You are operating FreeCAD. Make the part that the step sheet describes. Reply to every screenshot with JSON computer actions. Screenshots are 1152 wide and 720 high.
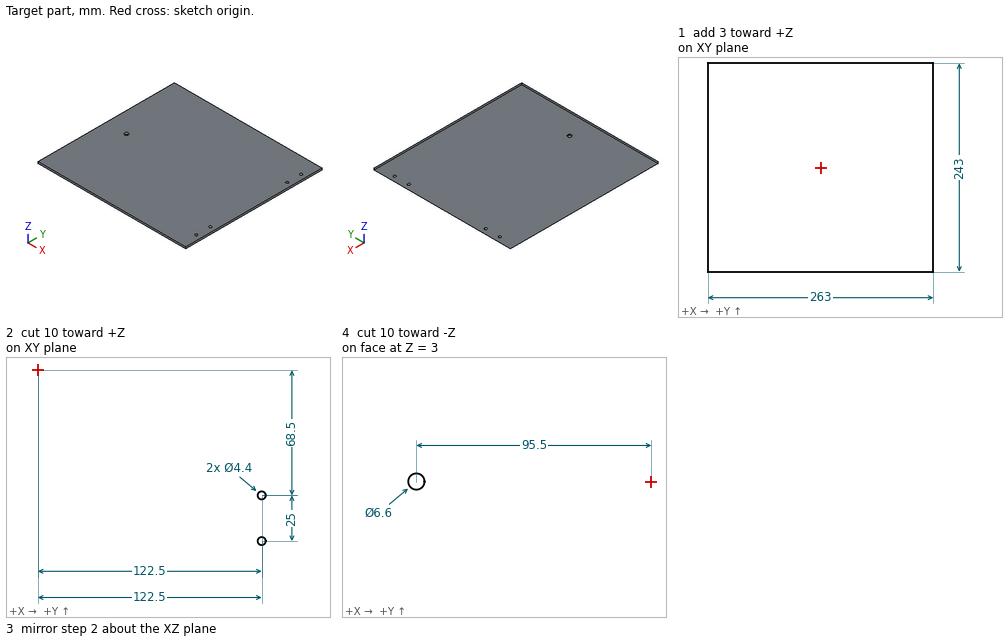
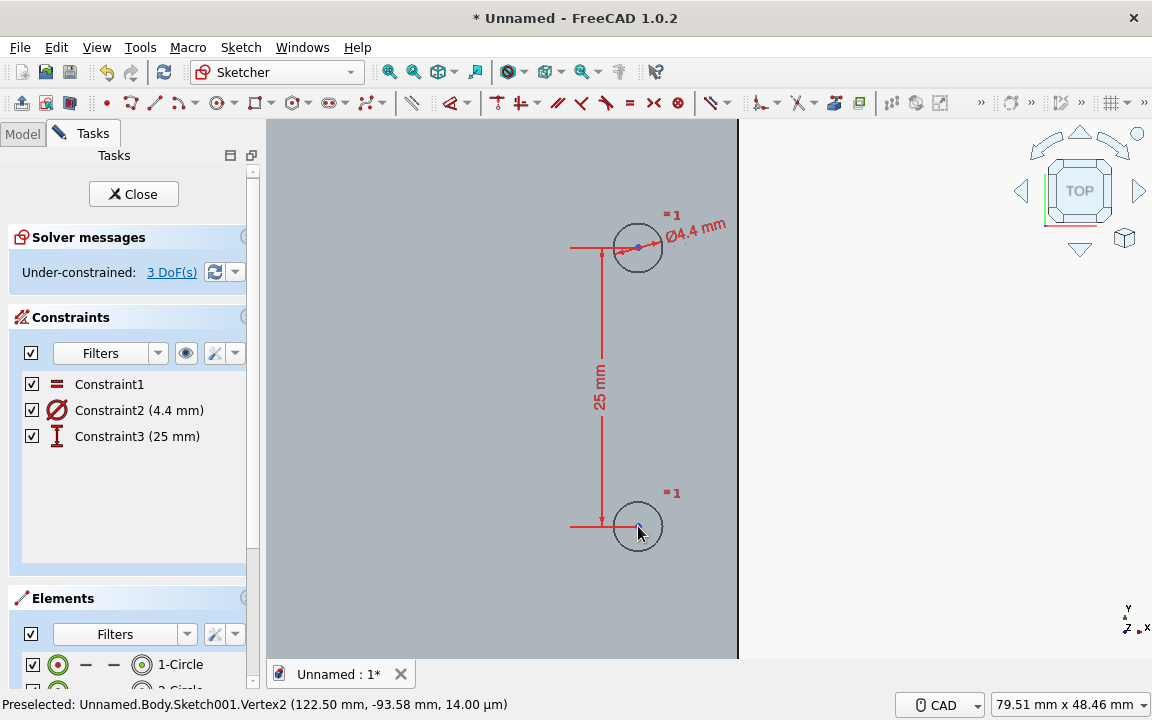
{"action": "left_click", "coordinate": [638, 248]}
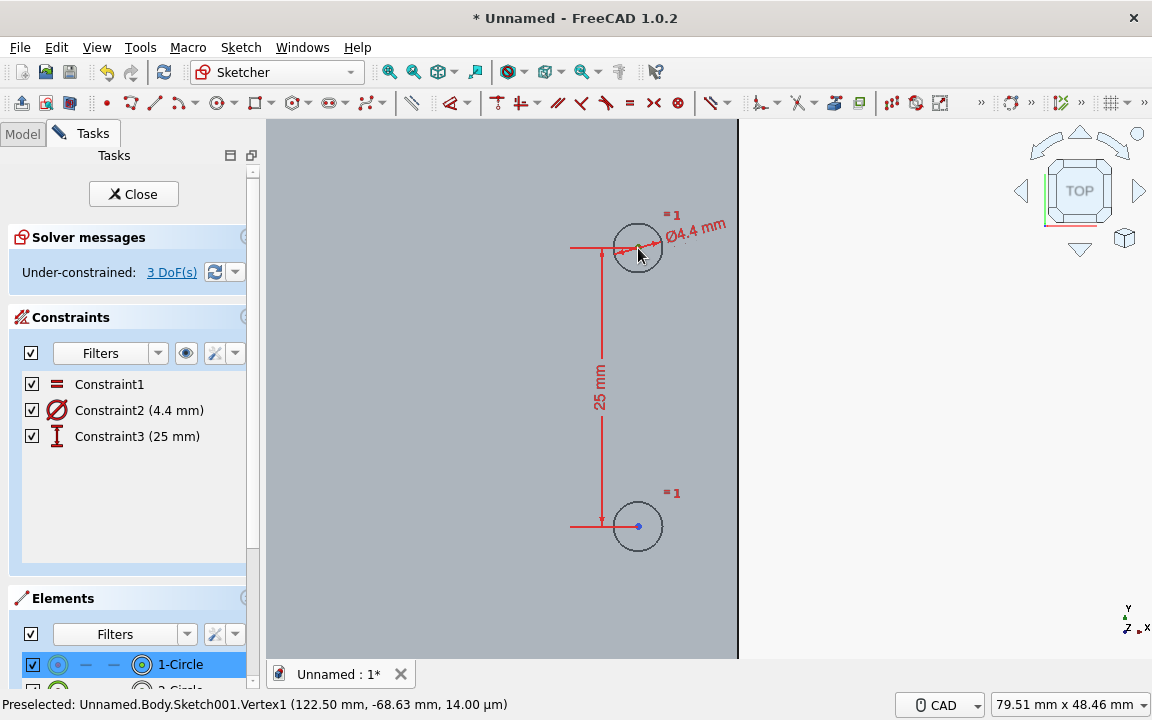
{"action": "key", "text": "i"}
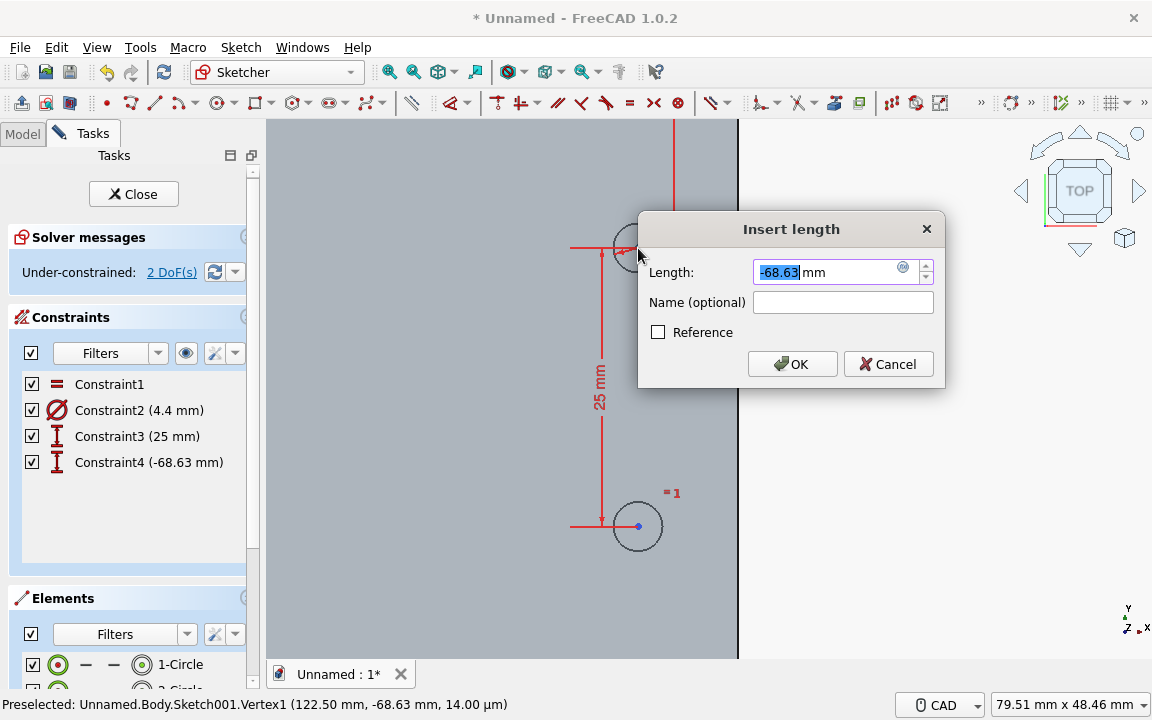
{"action": "type", "text": "-68.5"}
{"action": "key", "text": "Return"}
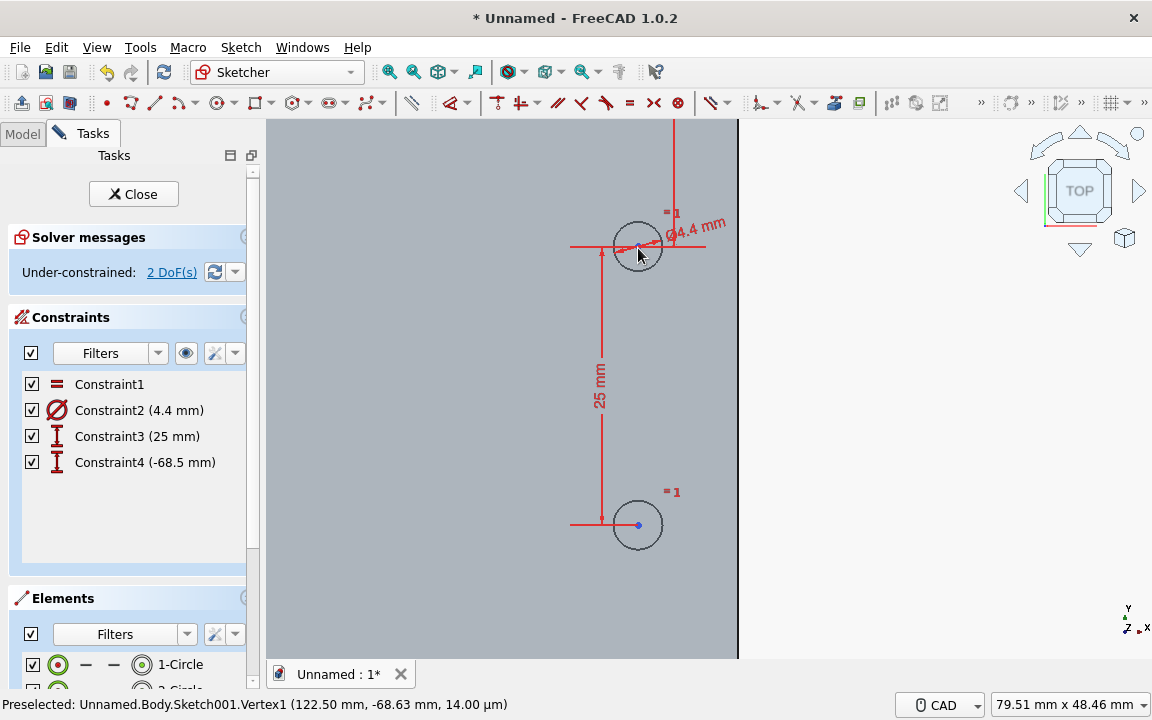
{"action": "left_click", "coordinate": [638, 247]}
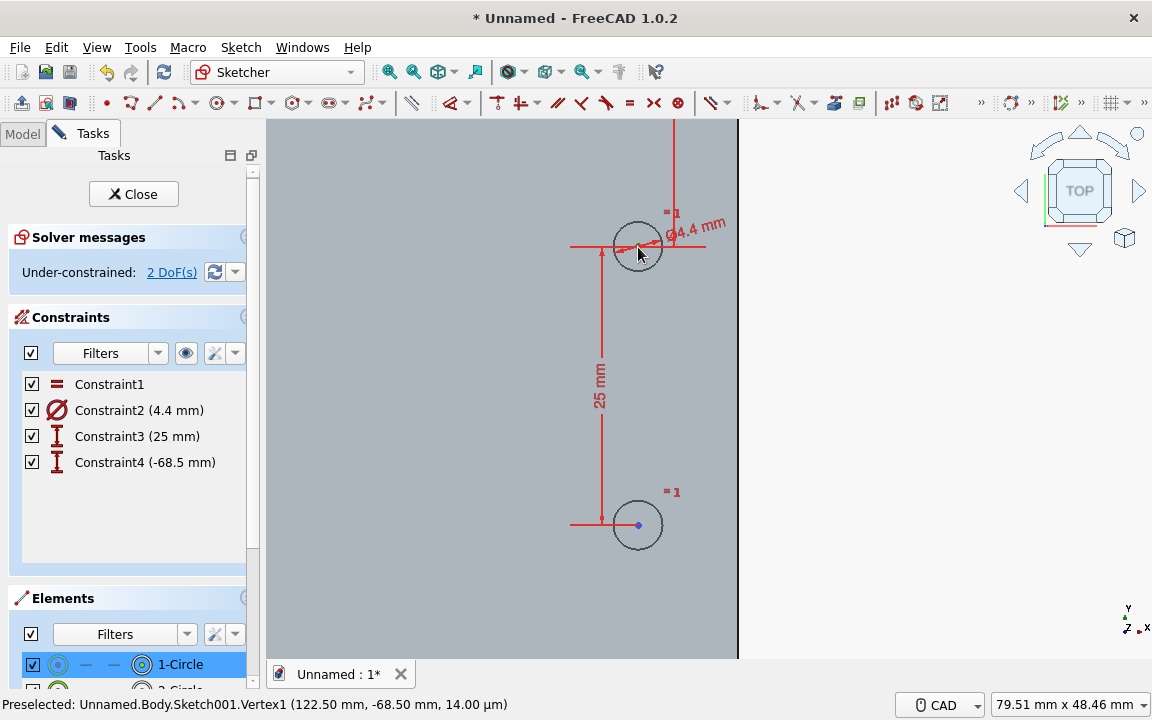
{"action": "left_click", "coordinate": [470, 104]}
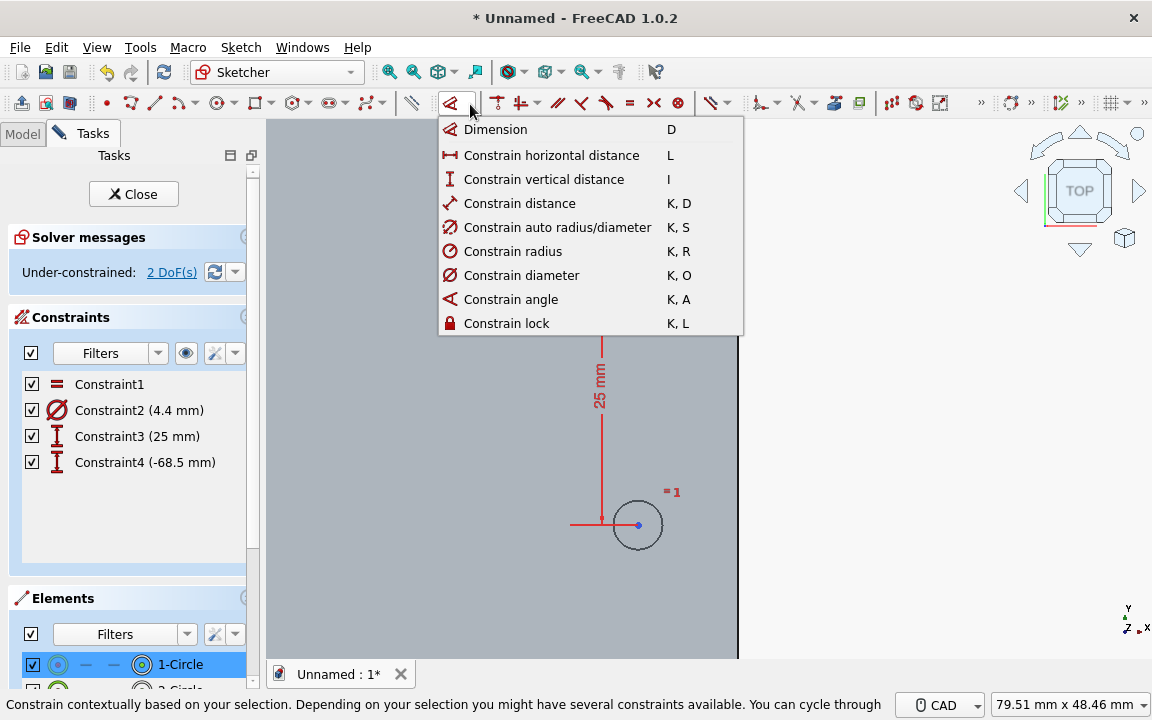
{"action": "left_click", "coordinate": [591, 155]}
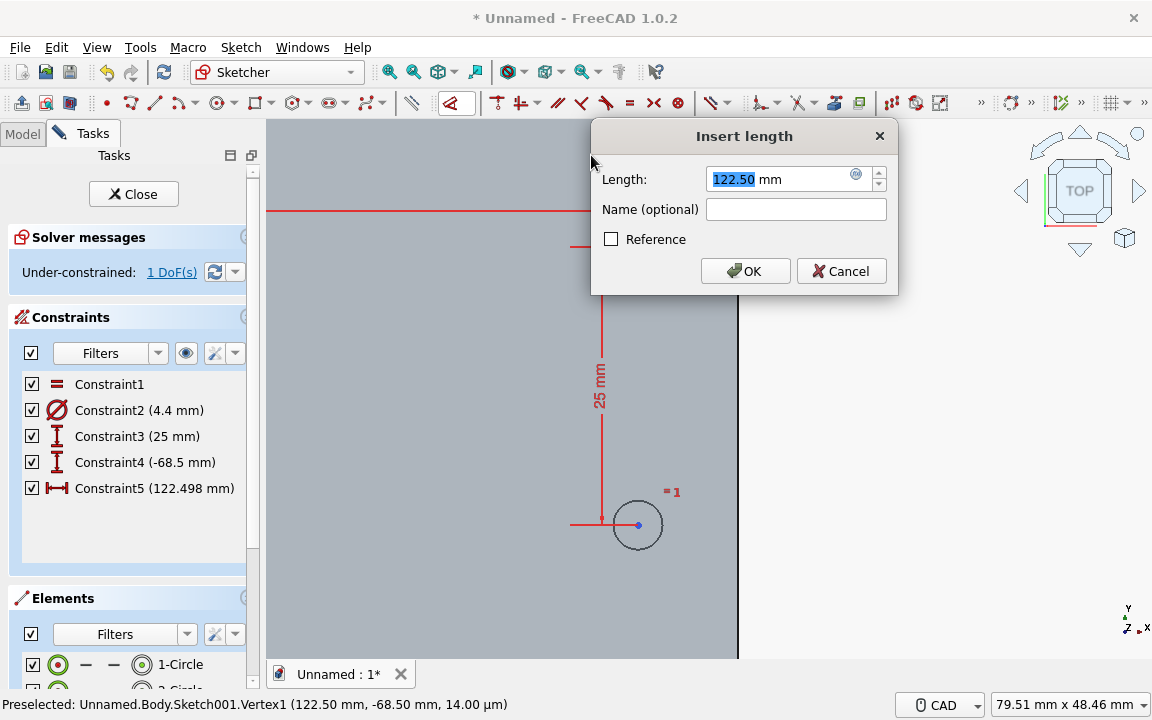
{"action": "type", "text": "122.5"}
{"action": "key", "text": "Return"}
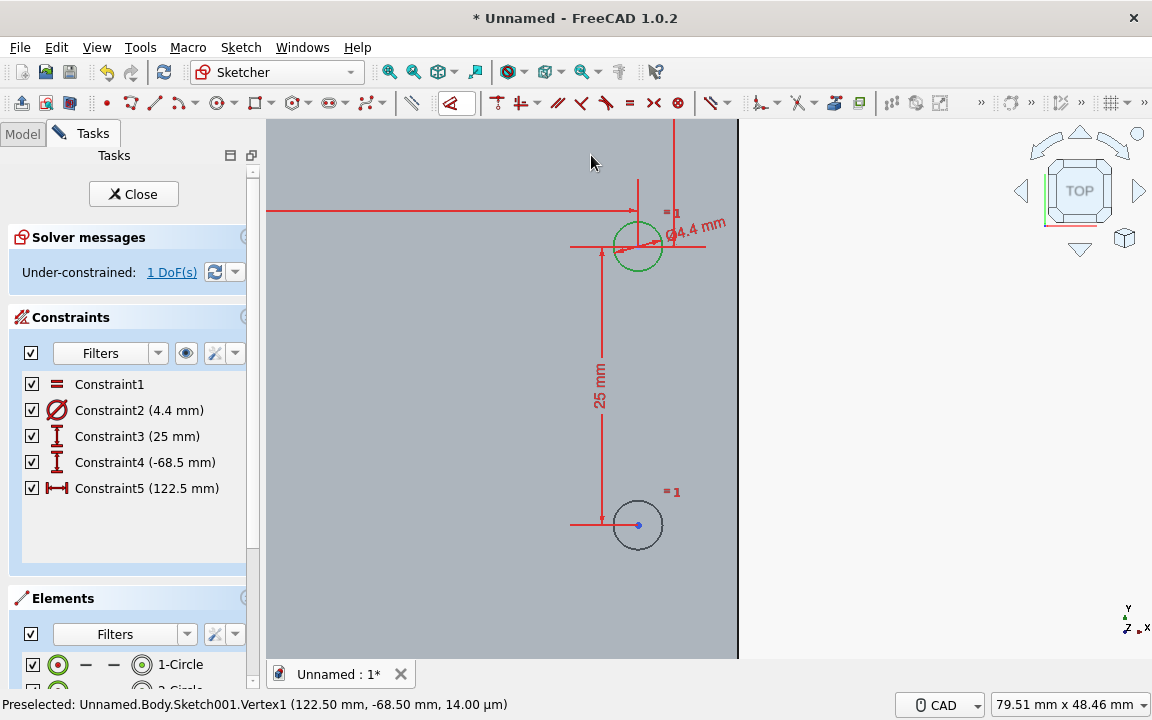
{"action": "left_click", "coordinate": [638, 525]}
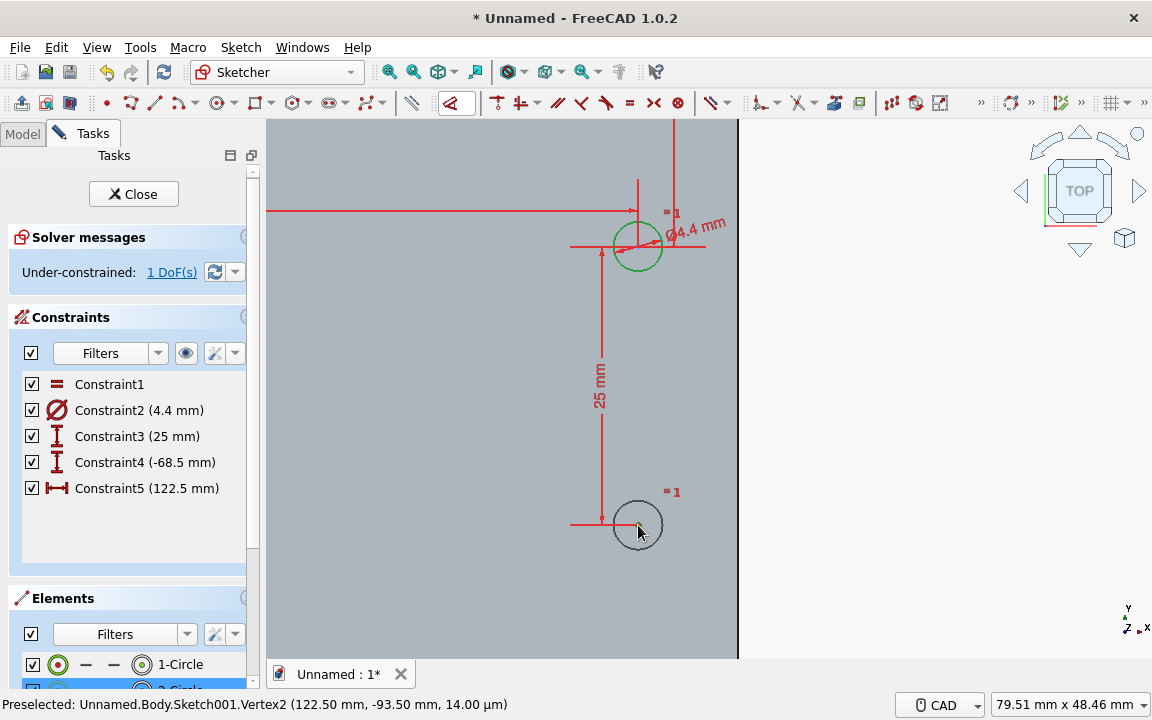
{"action": "key", "text": "l"}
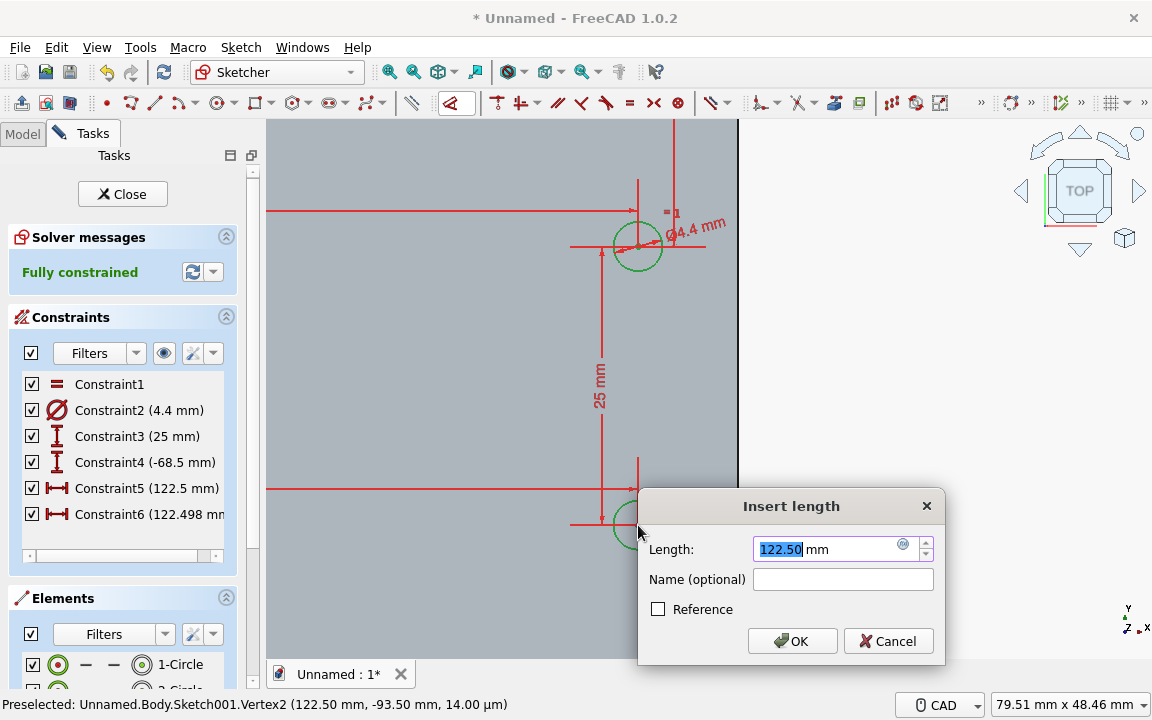
{"action": "type", "text": "122.5"}
{"action": "key", "text": "Return"}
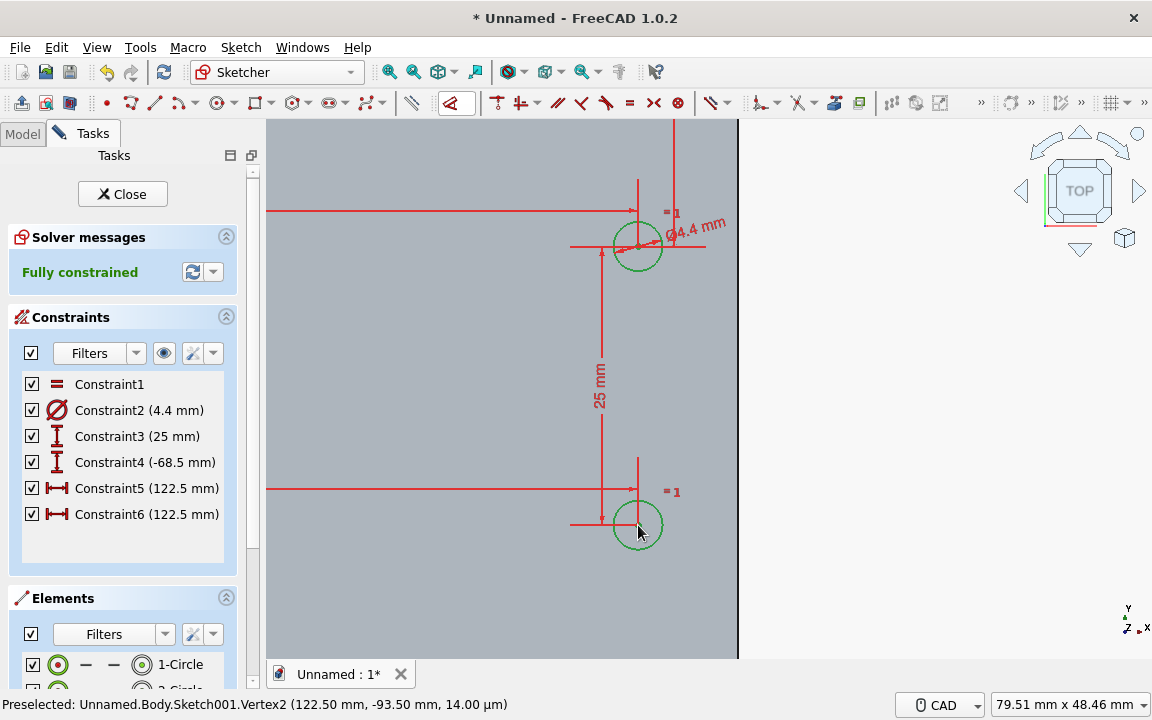
{"action": "left_click", "coordinate": [123, 194]}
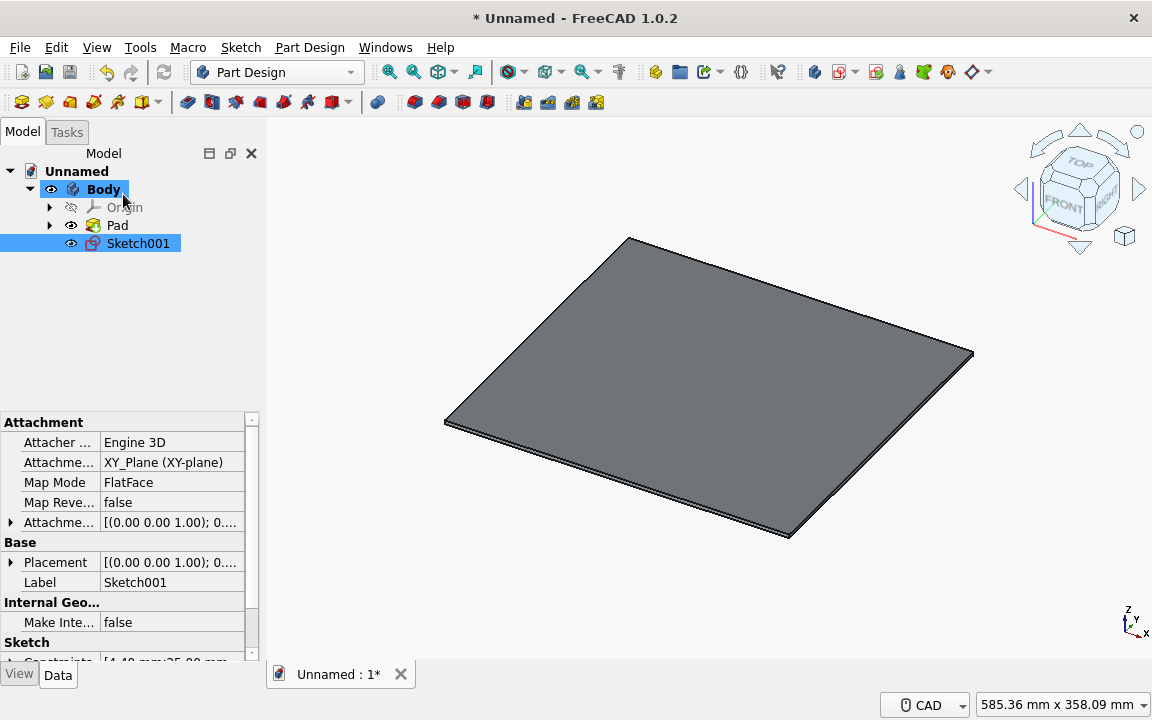
{"action": "left_click", "coordinate": [188, 102]}